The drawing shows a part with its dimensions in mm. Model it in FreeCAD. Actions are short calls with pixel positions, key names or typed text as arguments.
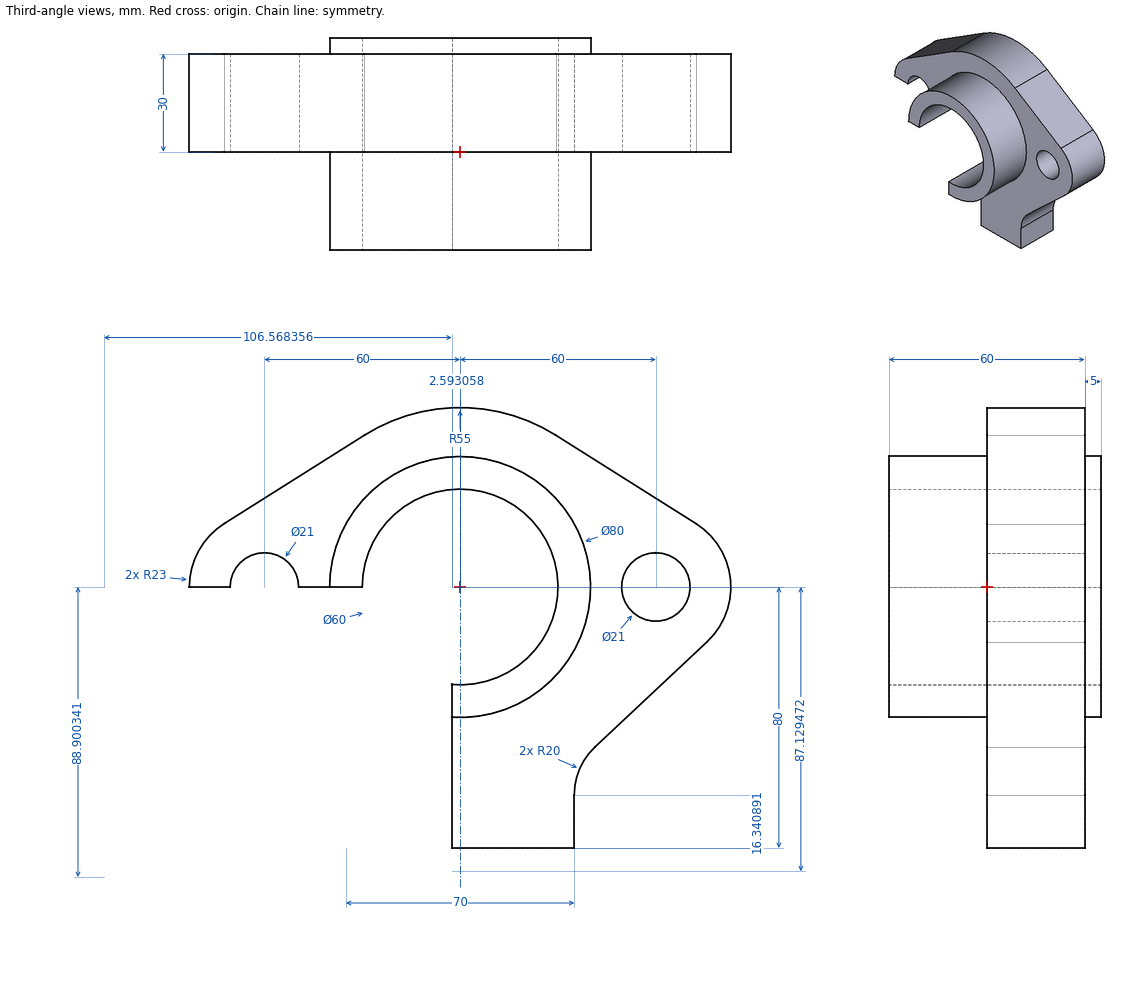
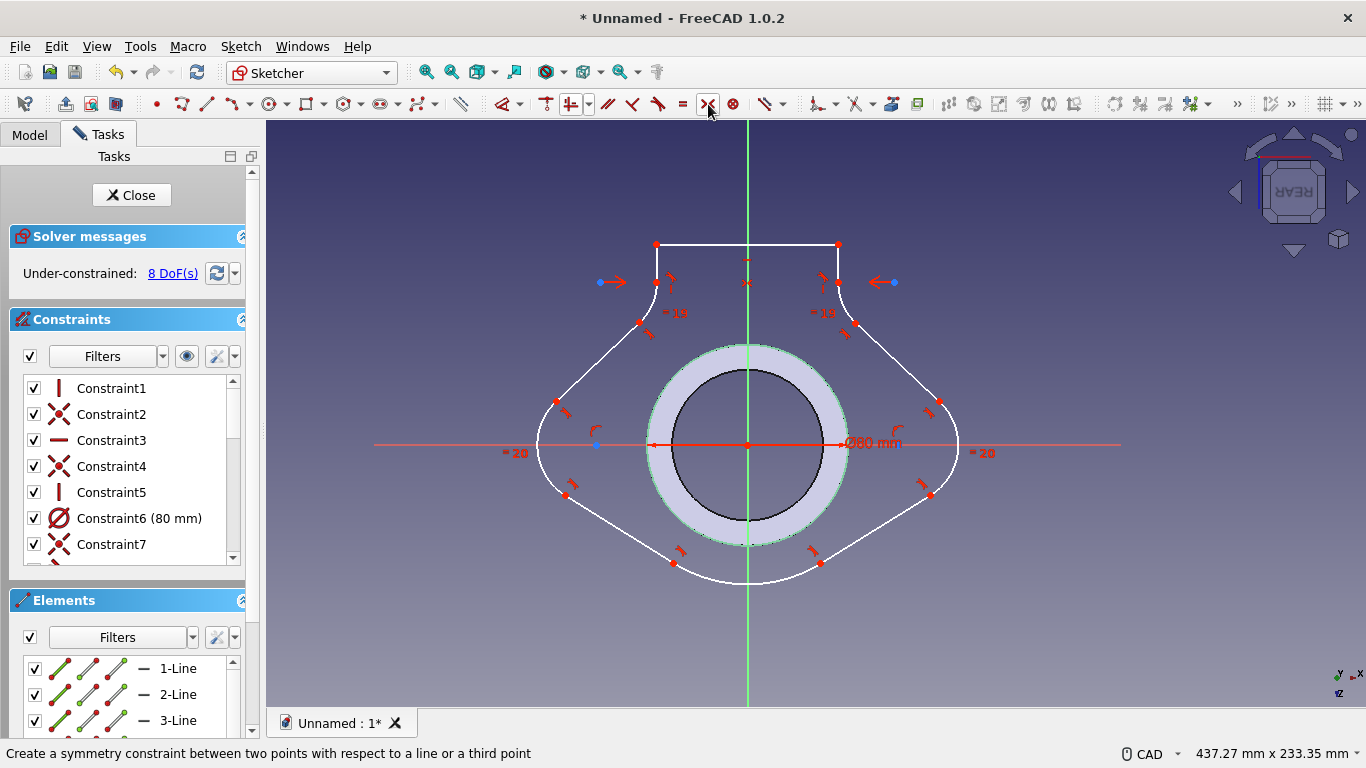
click(502, 104)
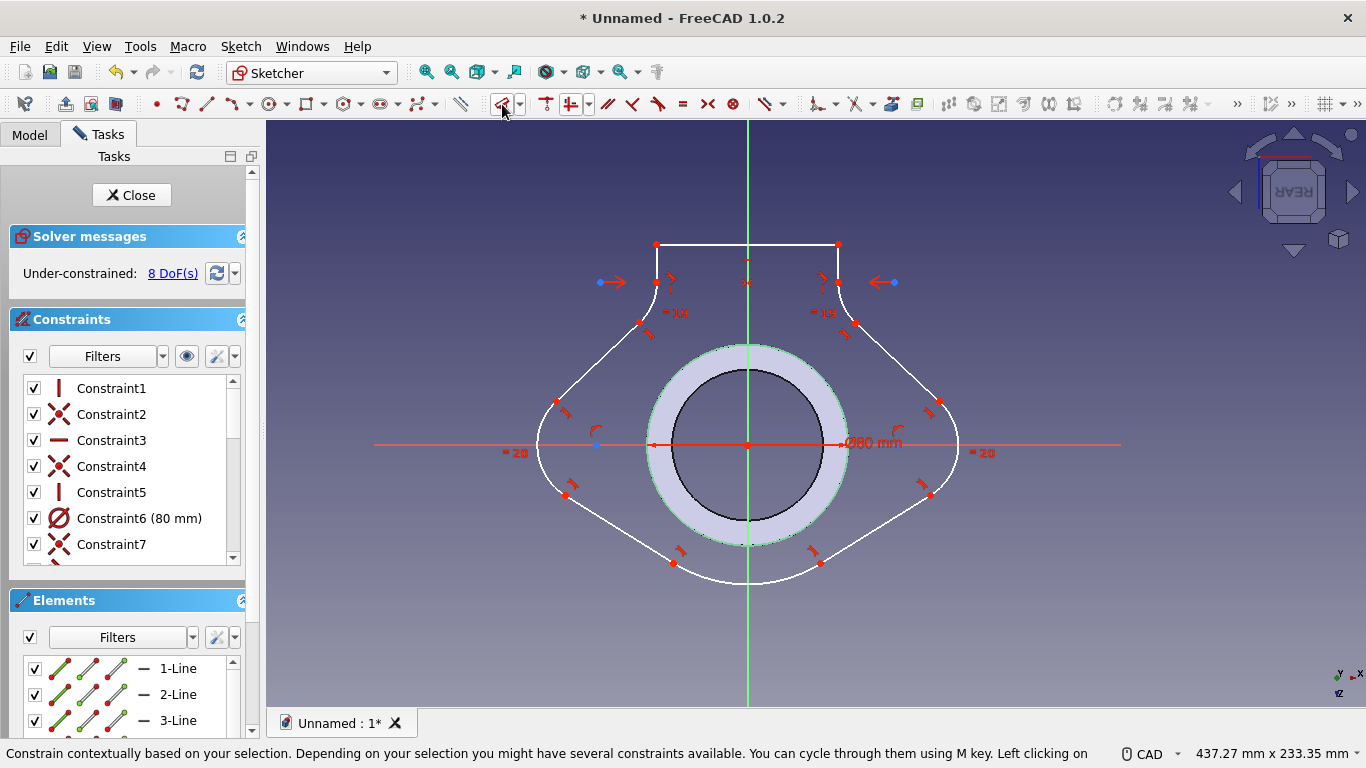
click(717, 581)
click(710, 612)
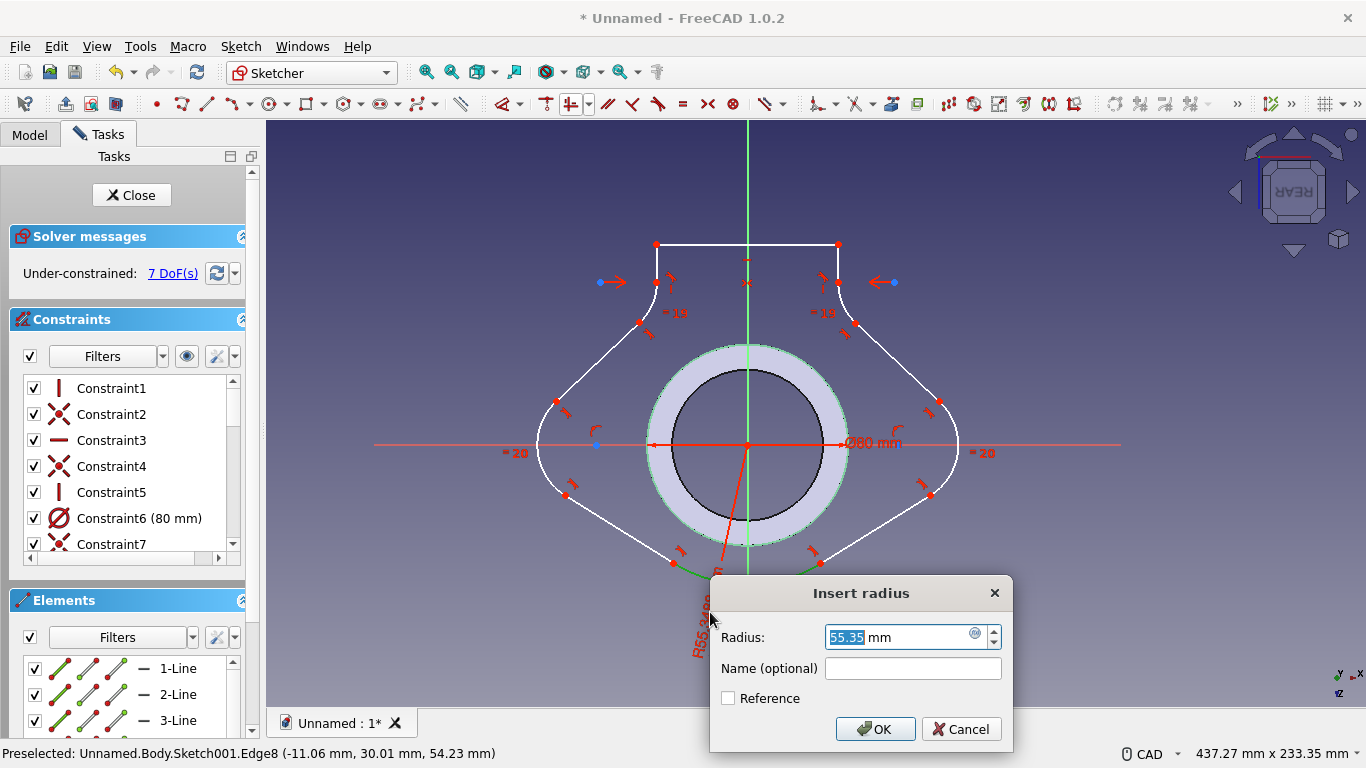
text(55)
key(Return)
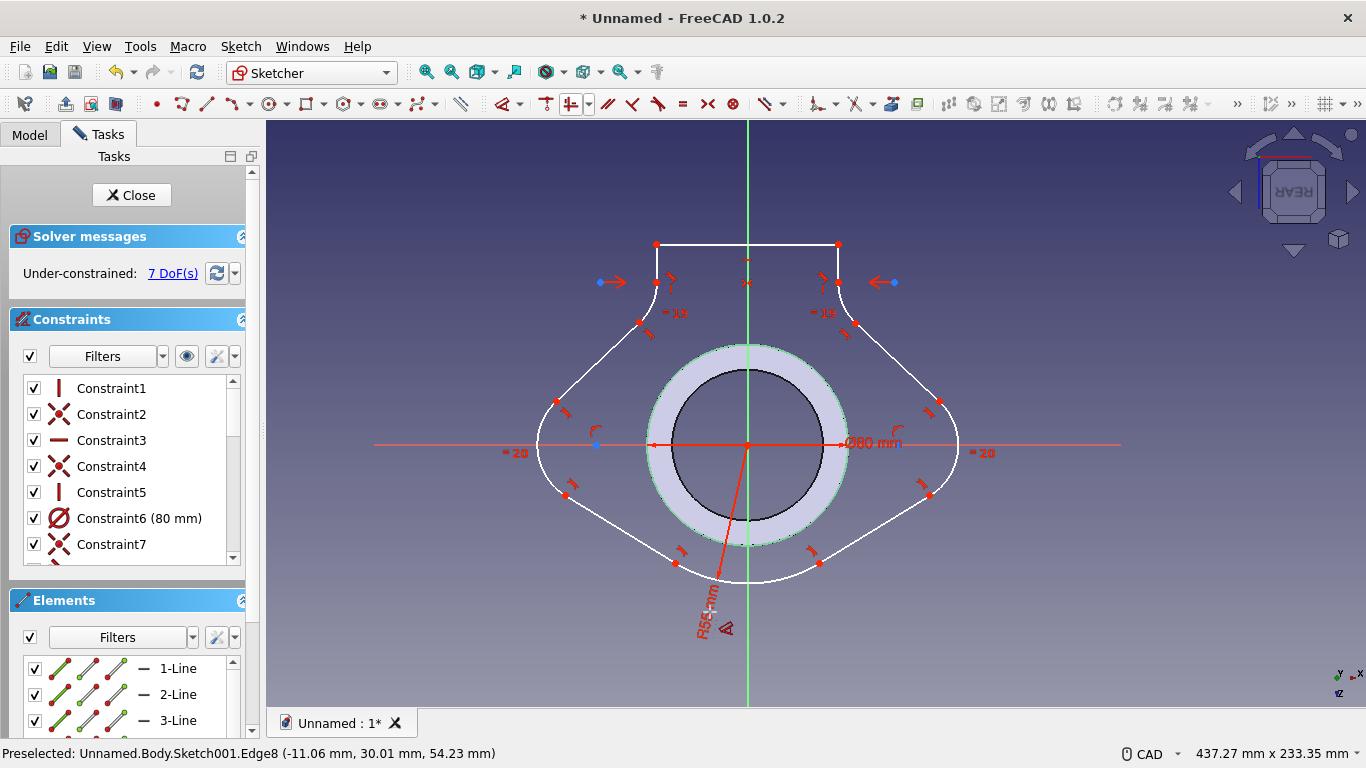
click(952, 472)
click(981, 486)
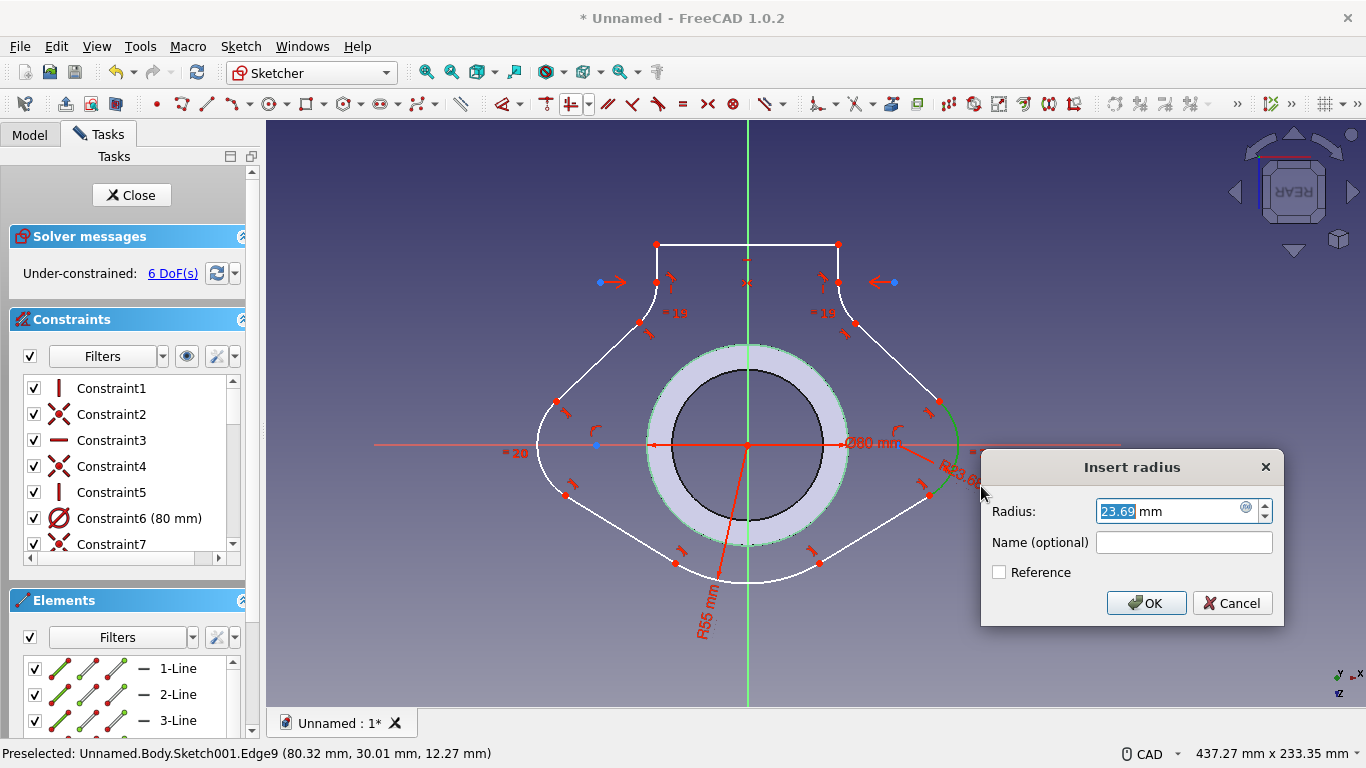
text(23)
key(Return)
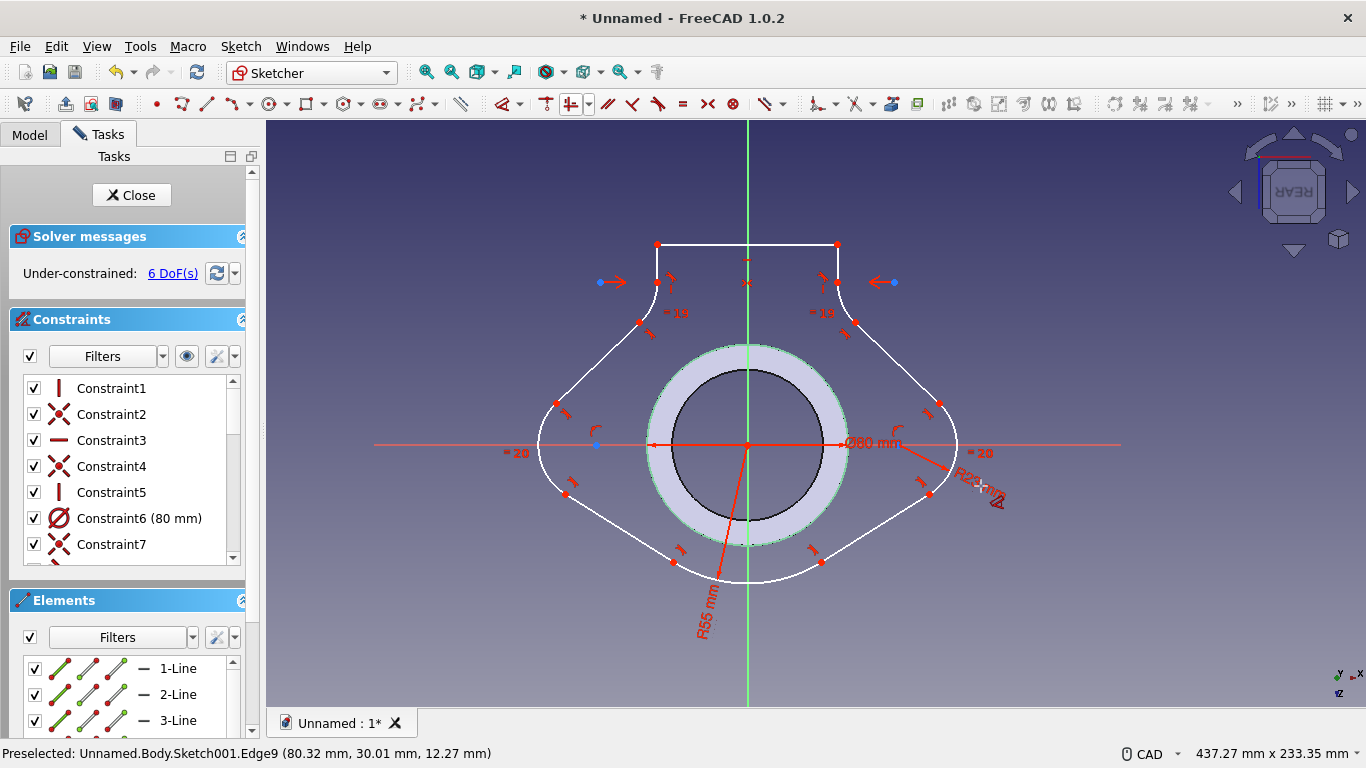
click(840, 296)
click(809, 304)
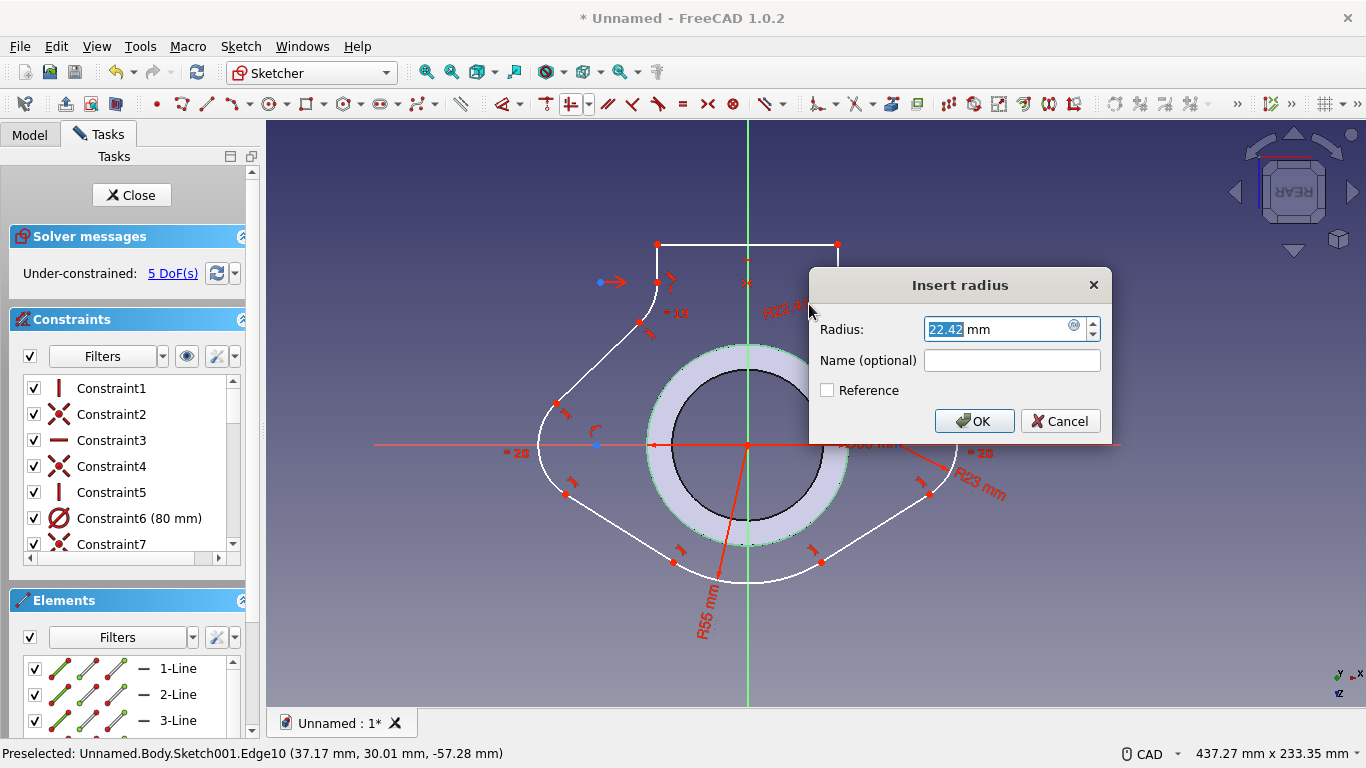
text(20)
key(Return)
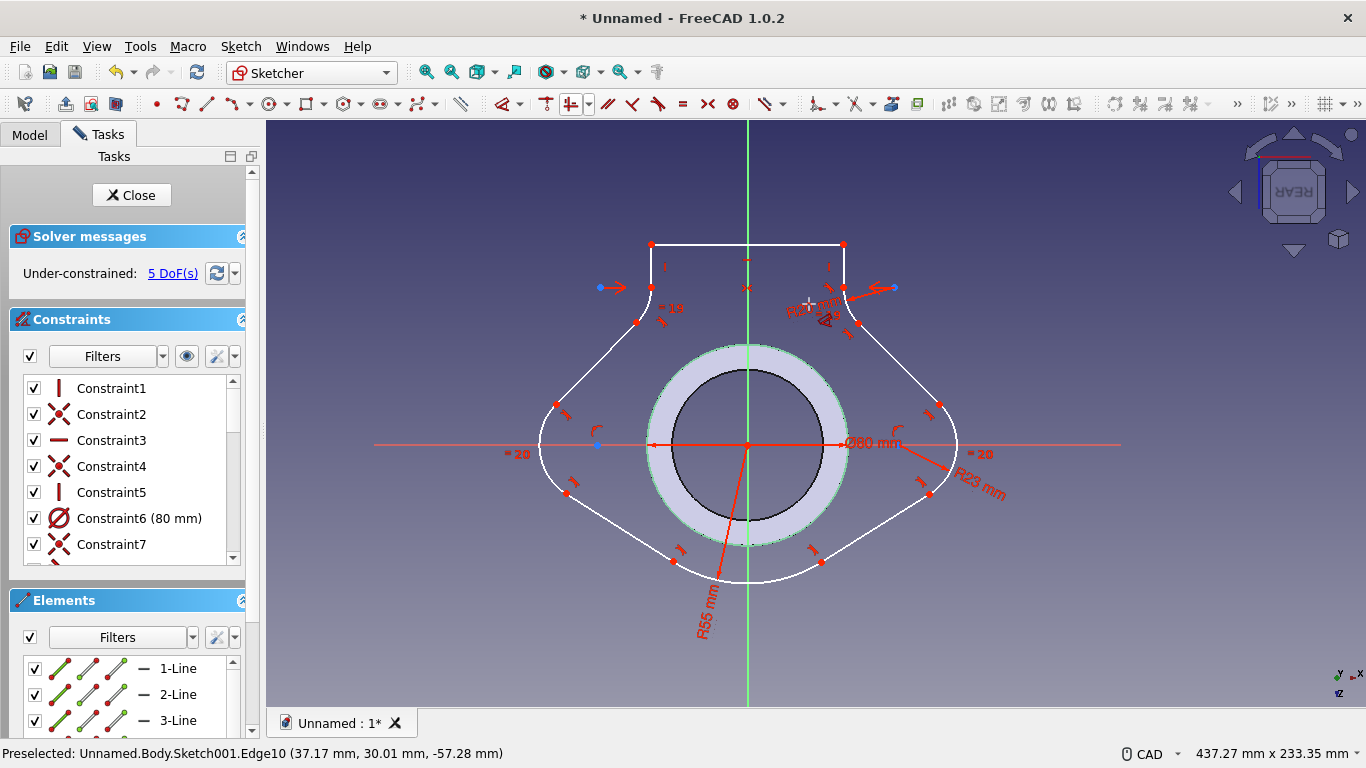
click(786, 245)
click(703, 211)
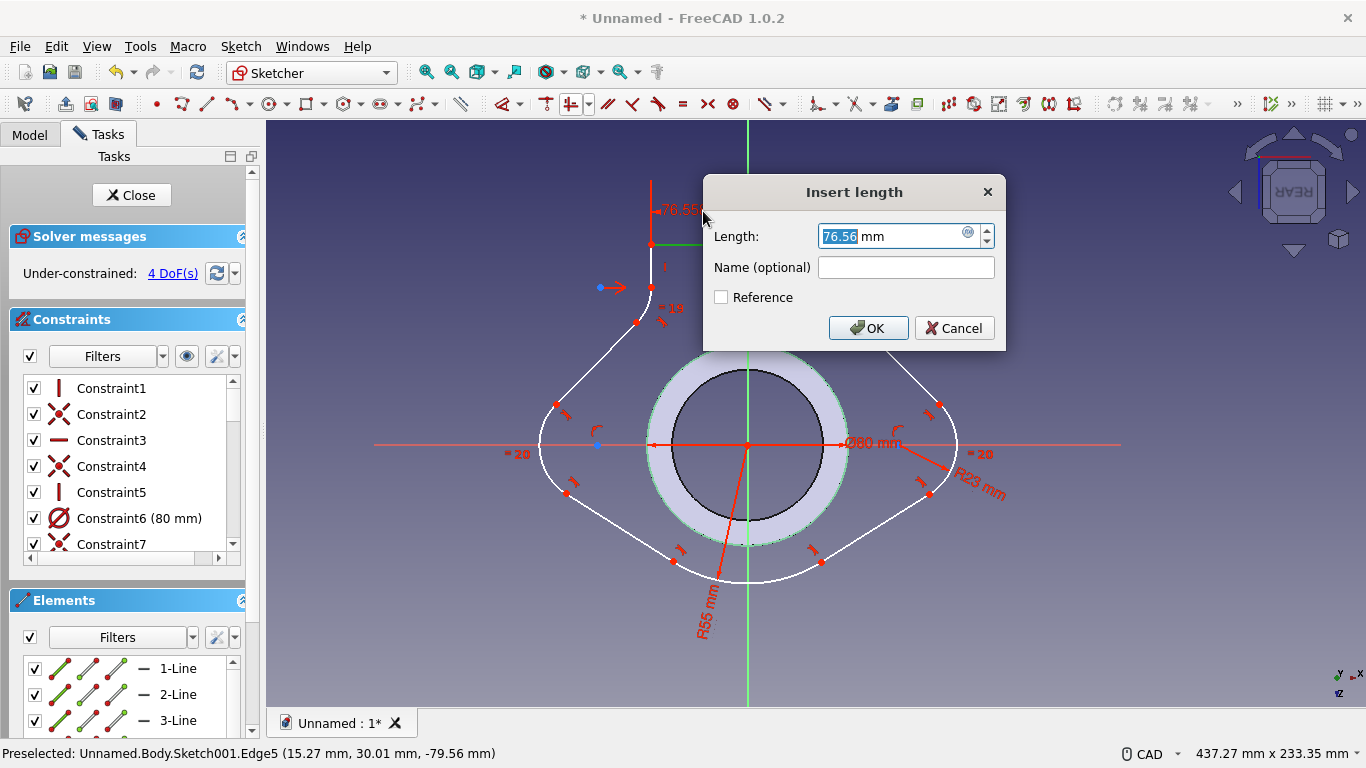
text(70)
key(Return)